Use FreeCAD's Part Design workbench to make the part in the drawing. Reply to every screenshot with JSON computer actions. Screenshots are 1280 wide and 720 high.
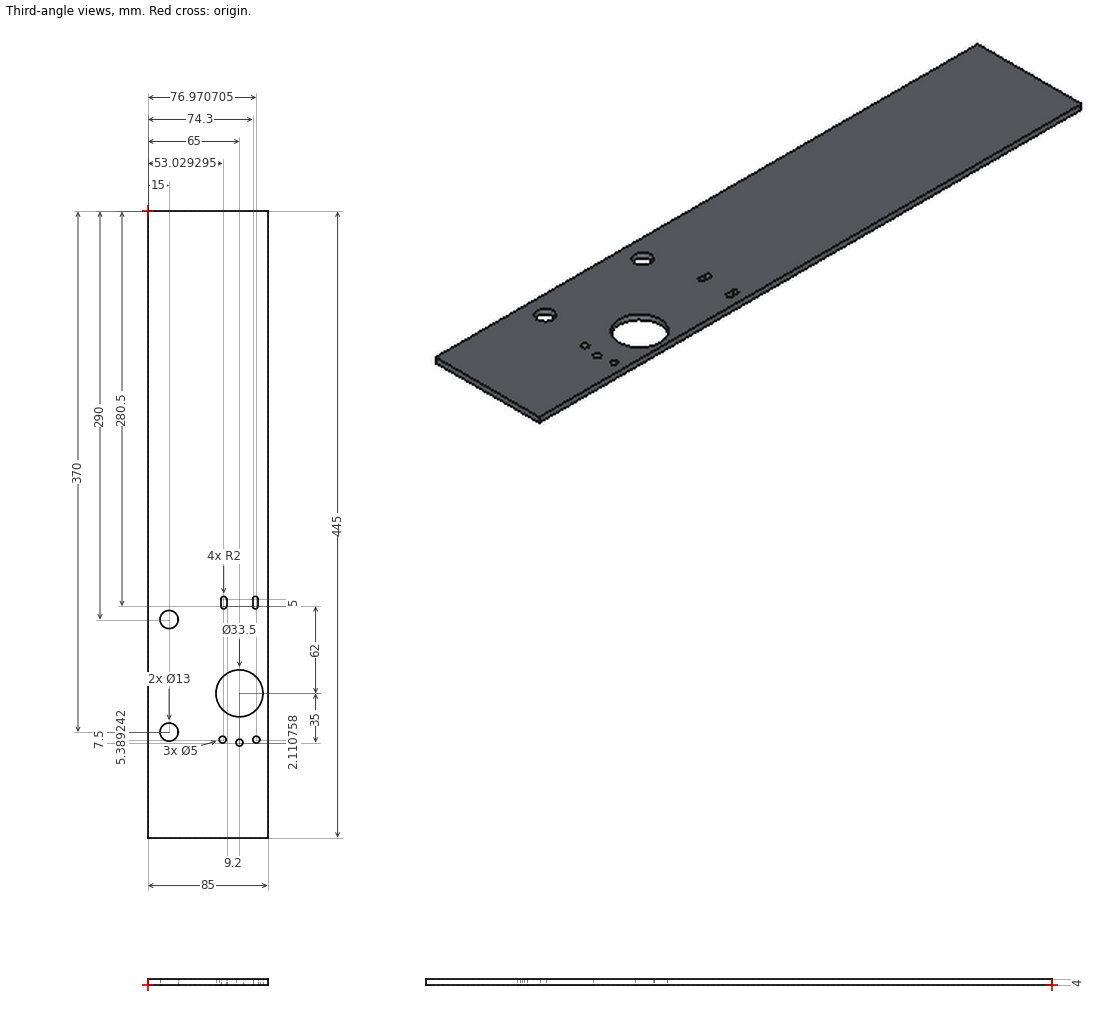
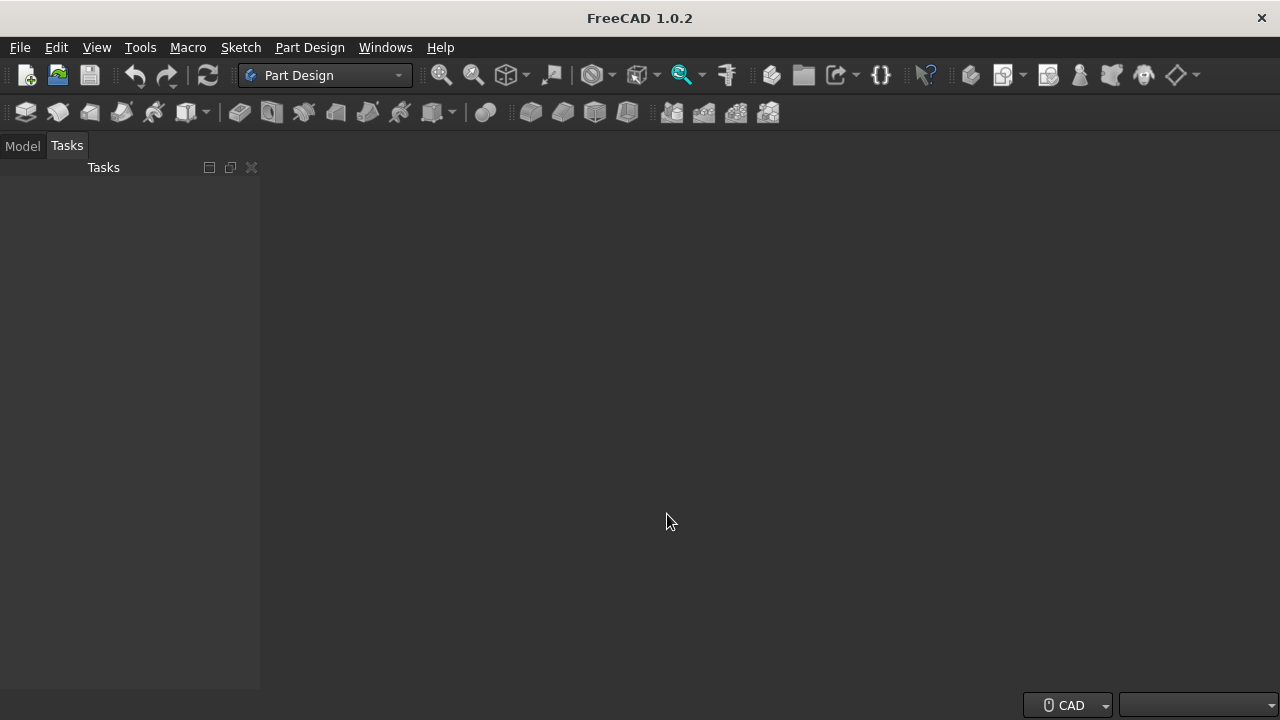
{"action": "left_click", "coordinate": [26, 76]}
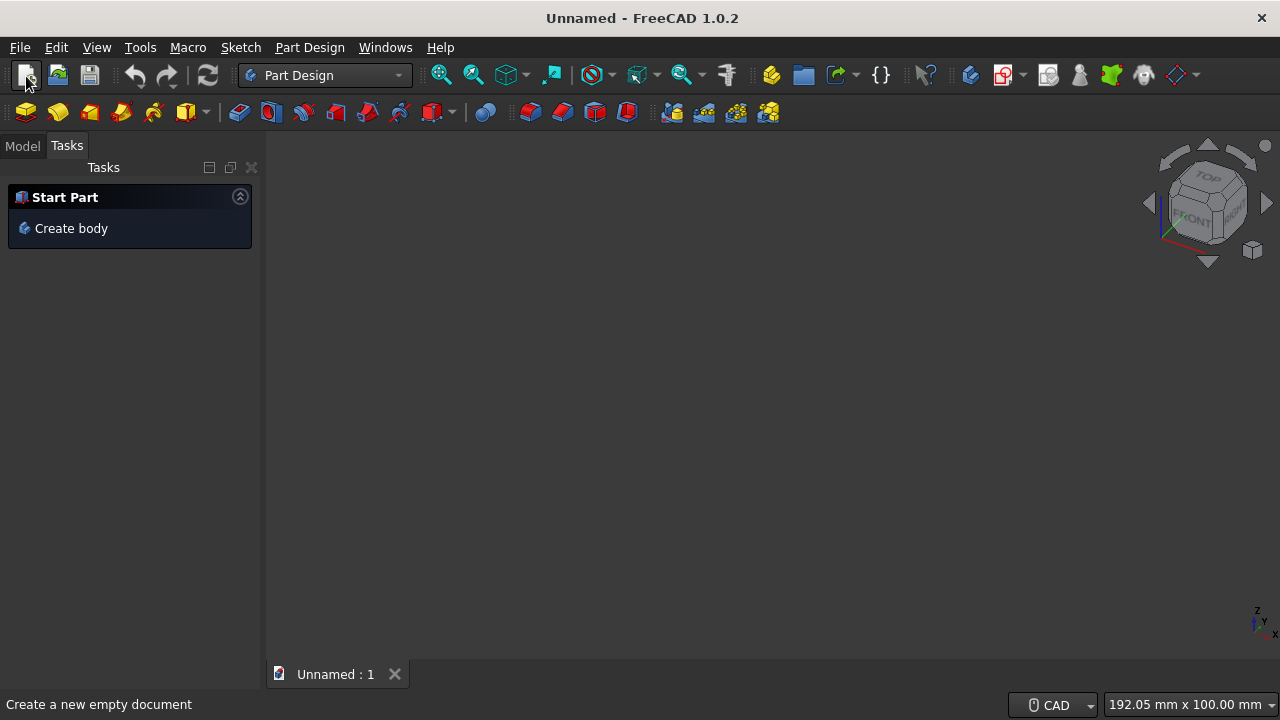
{"action": "left_click", "coordinate": [1004, 76]}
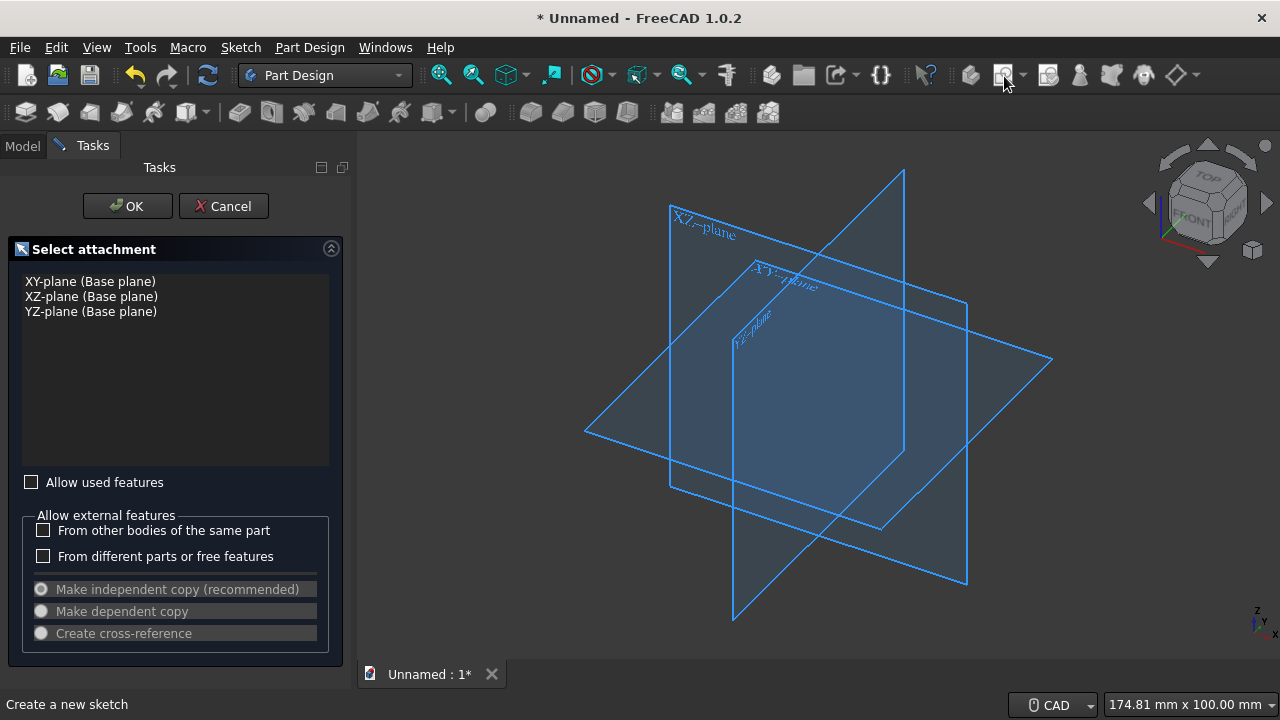
{"action": "left_click", "coordinate": [82, 282]}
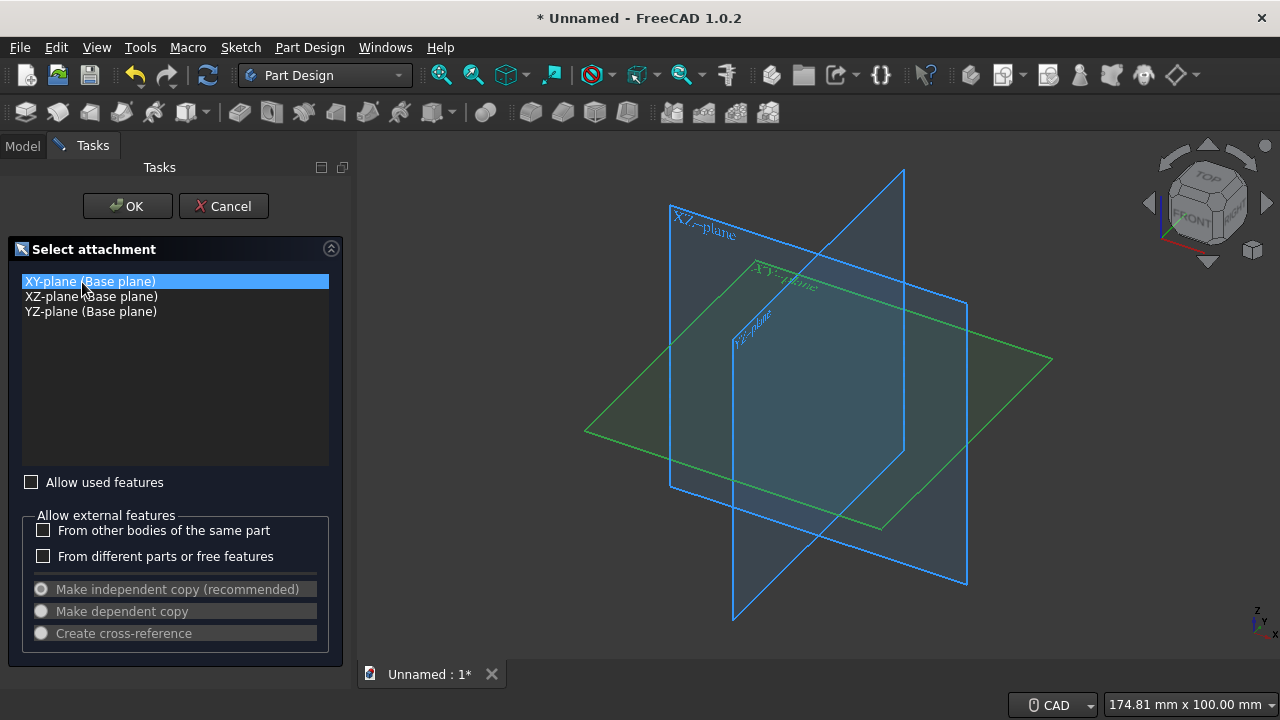
{"action": "left_click", "coordinate": [128, 206]}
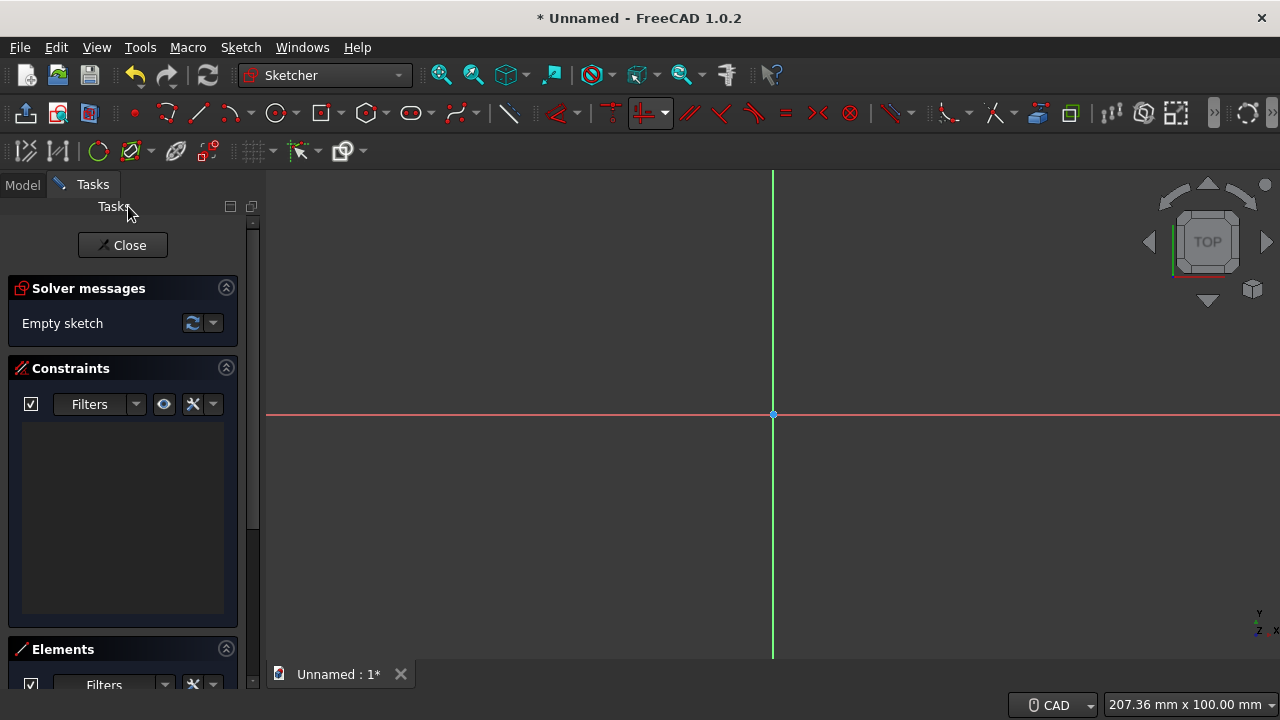
{"action": "scroll", "coordinate": [661, 244], "scroll_direction": "down", "scroll_amount": 10}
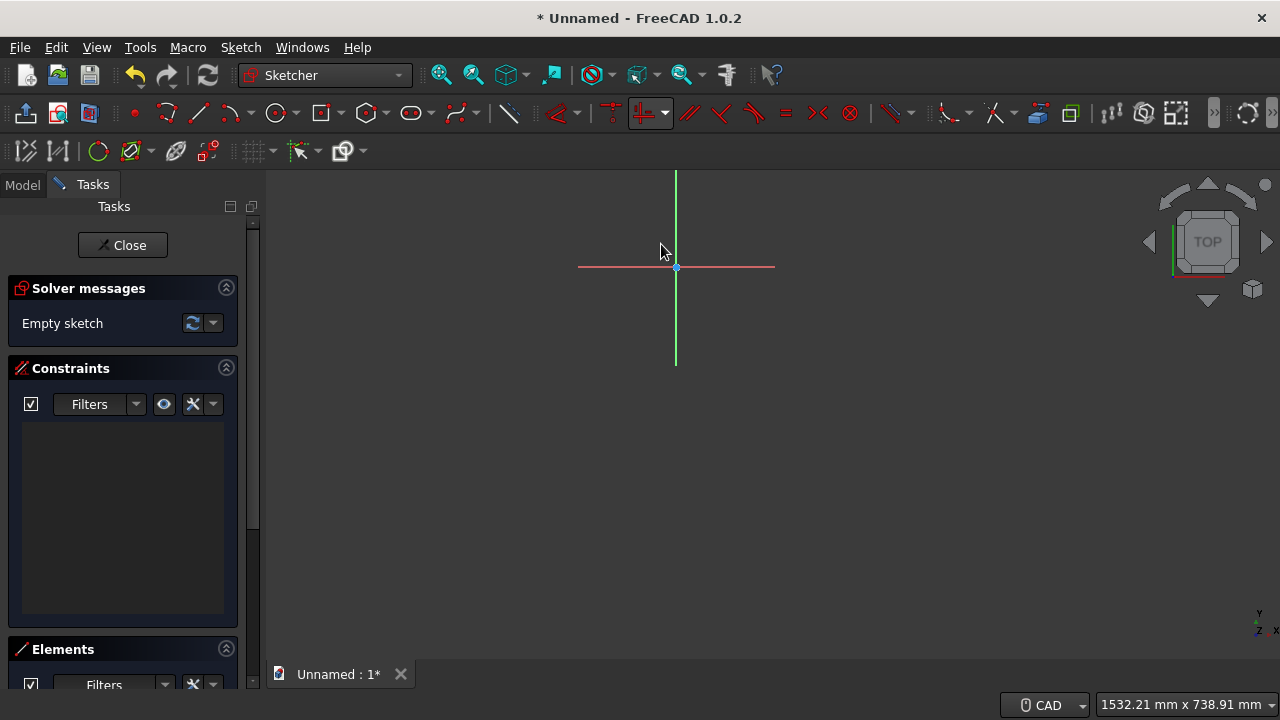
{"action": "key", "text": "g r"}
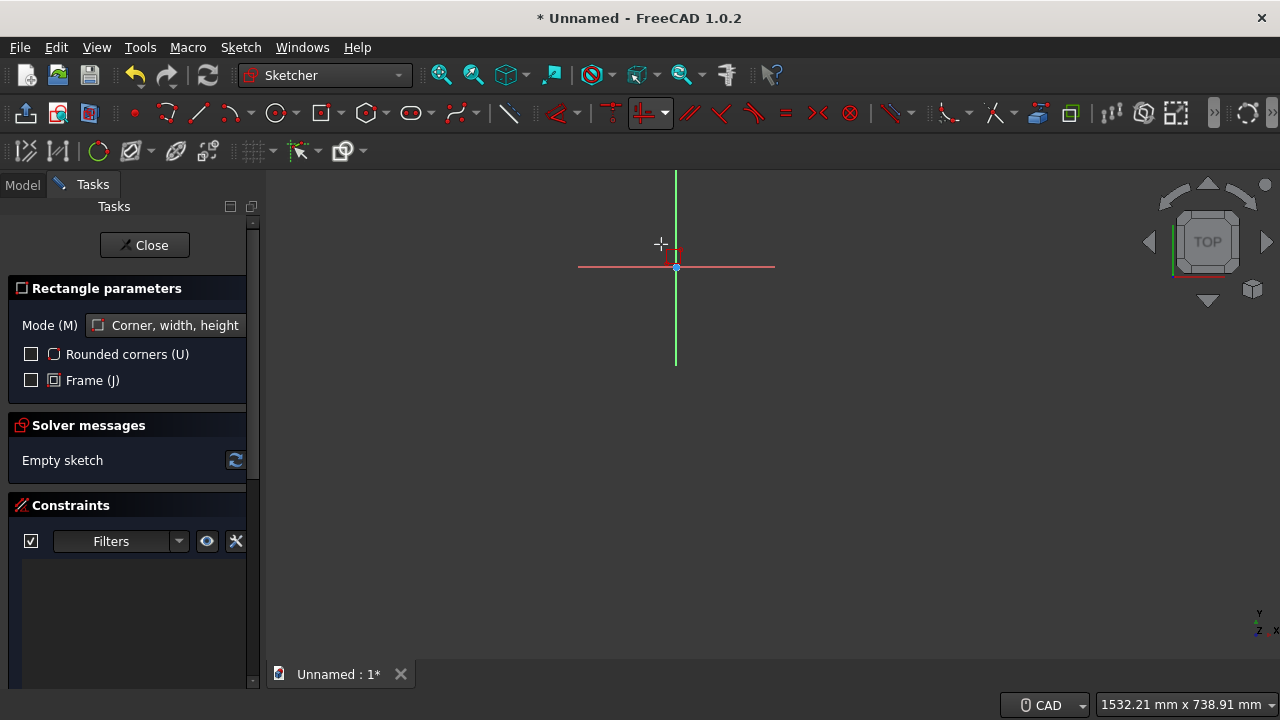
{"action": "left_click", "coordinate": [676, 267]}
{"action": "mouse_move", "coordinate": [733, 562]}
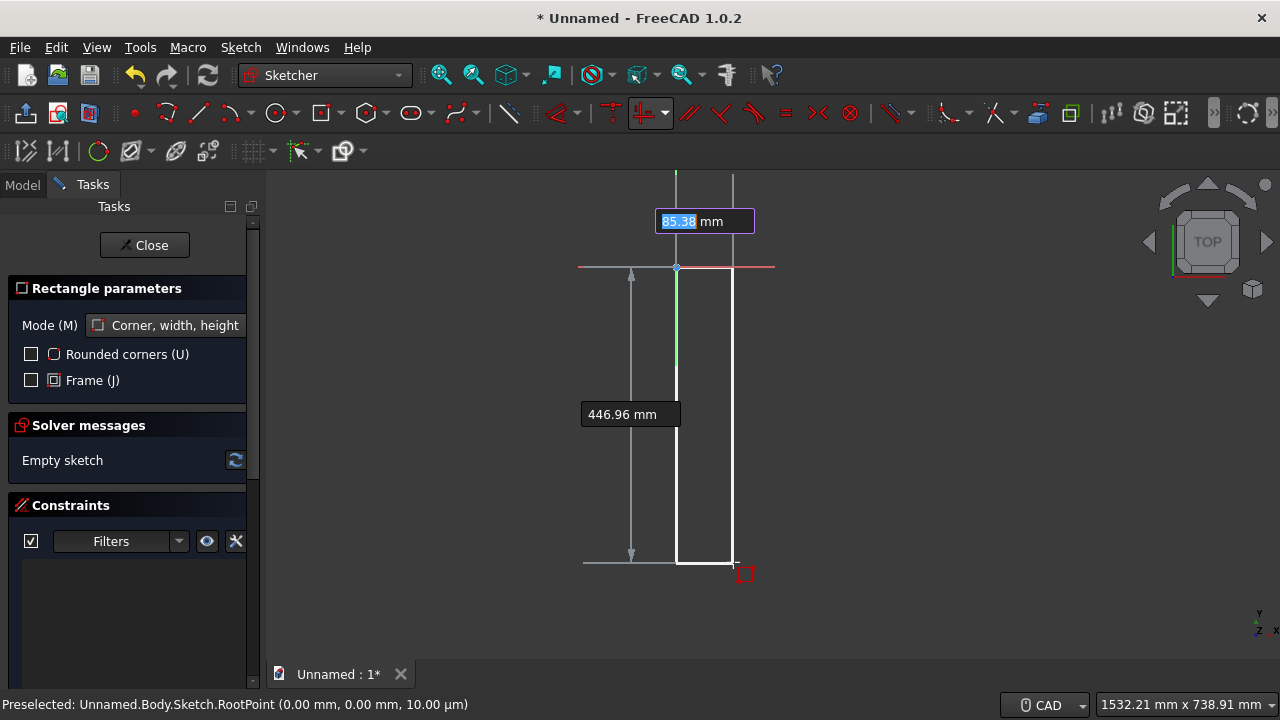
{"action": "type", "text": "85"}
{"action": "key", "text": "Tab"}
{"action": "type", "text": "445"}
{"action": "key", "text": "Return"}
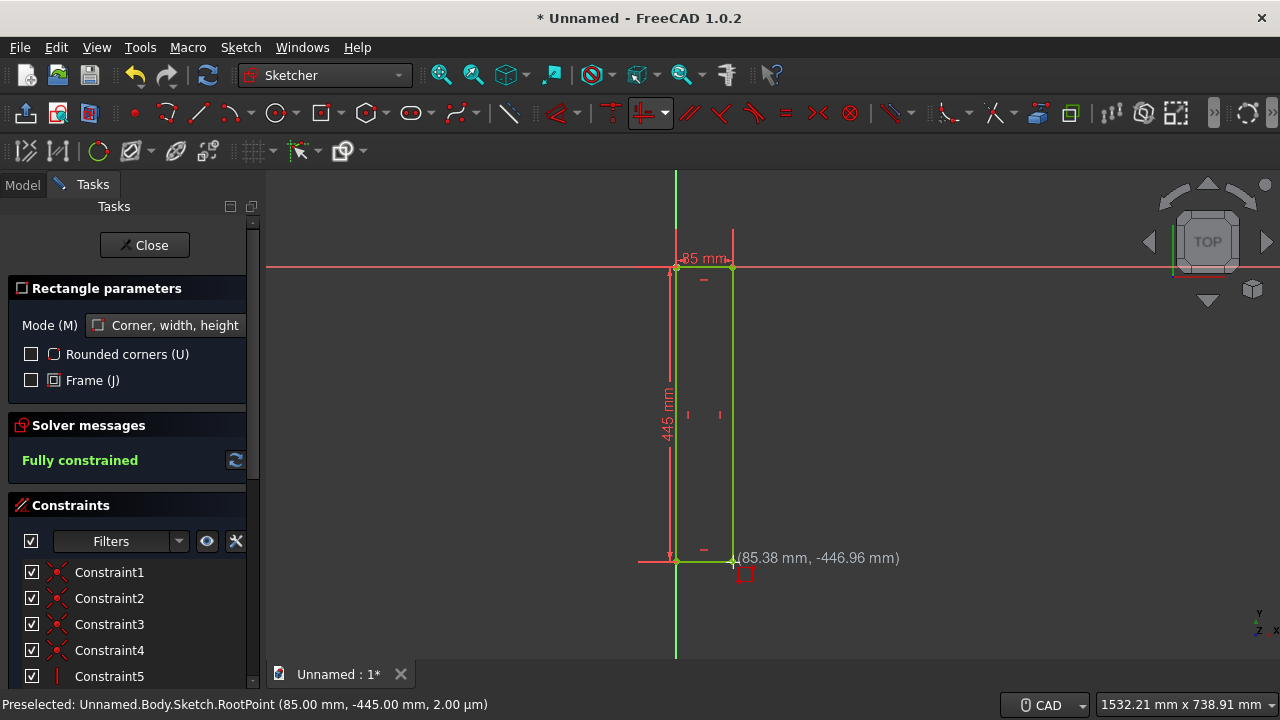
{"action": "left_click", "coordinate": [412, 114]}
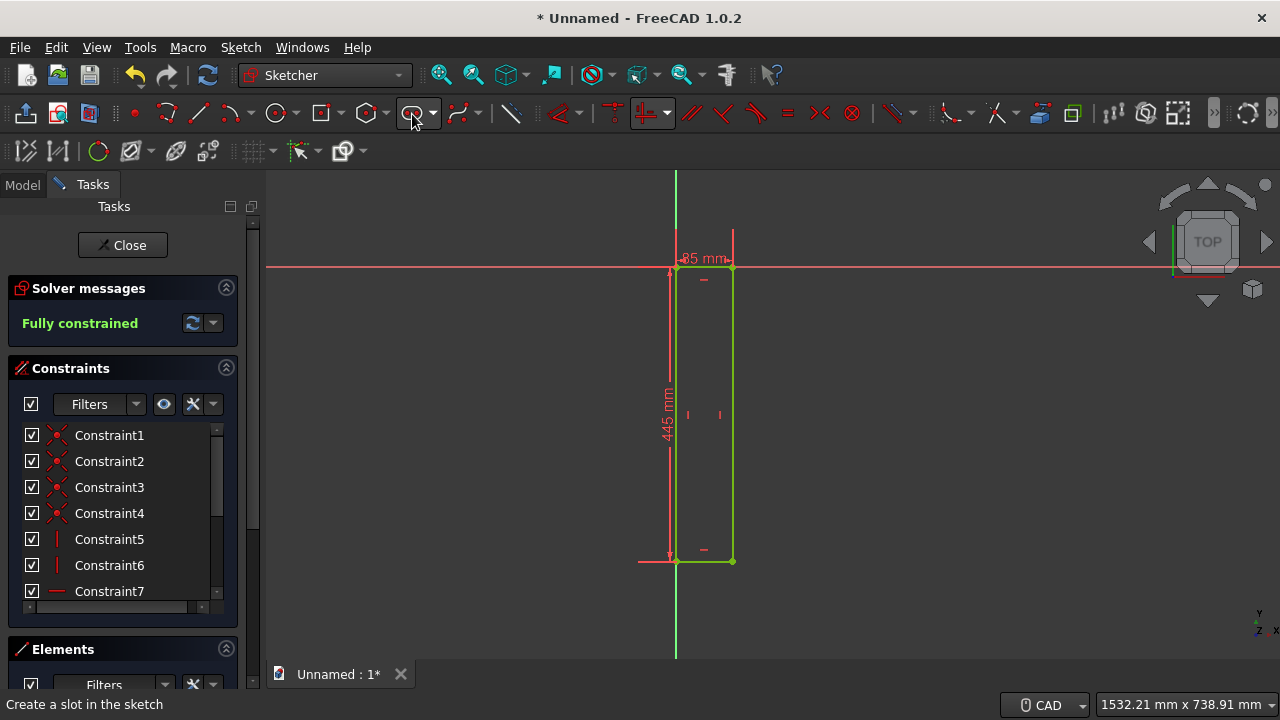
{"action": "scroll", "coordinate": [712, 453], "scroll_direction": "up", "scroll_amount": 15}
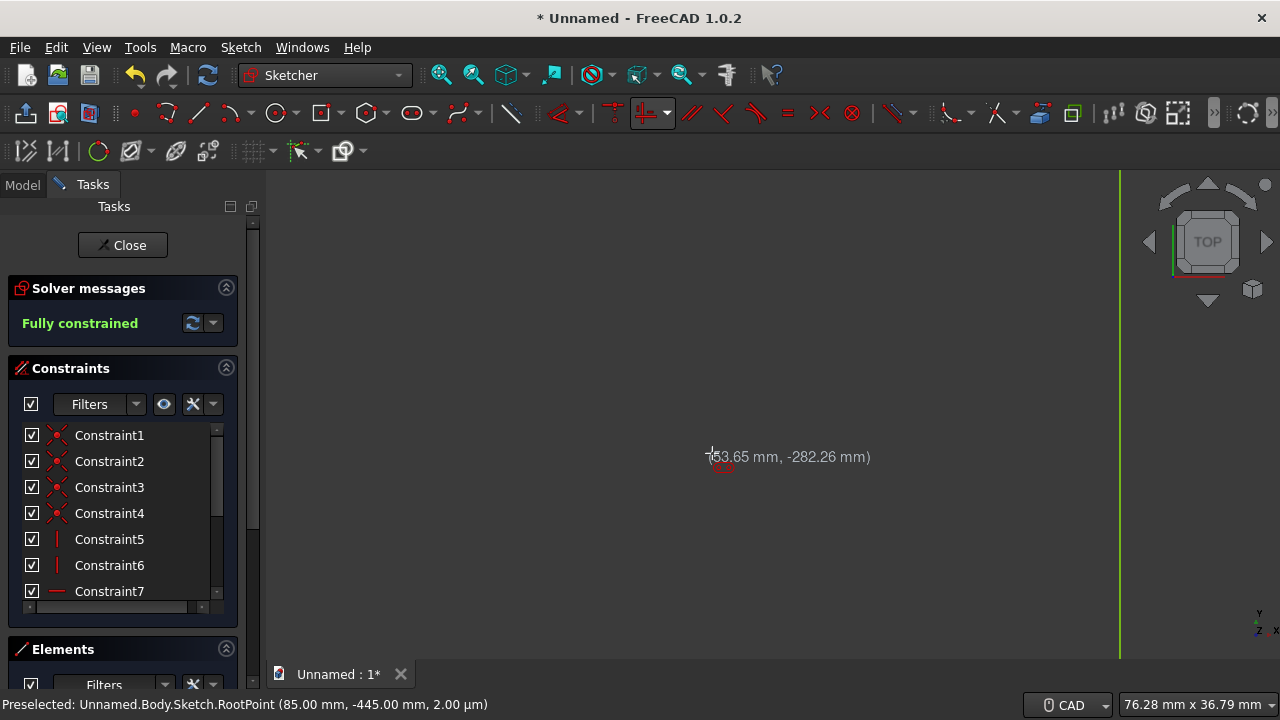
{"action": "scroll", "coordinate": [712, 454], "scroll_direction": "down", "scroll_amount": 15}